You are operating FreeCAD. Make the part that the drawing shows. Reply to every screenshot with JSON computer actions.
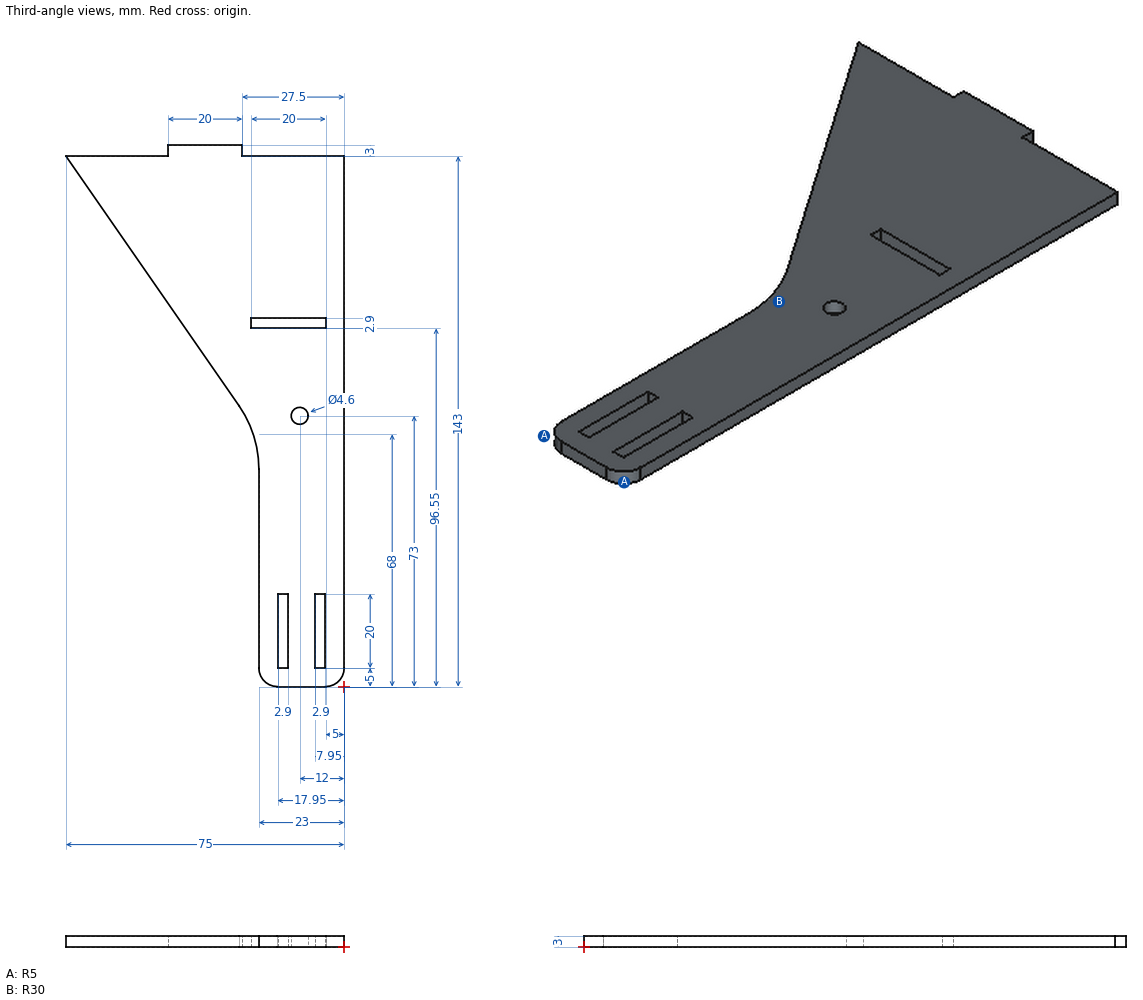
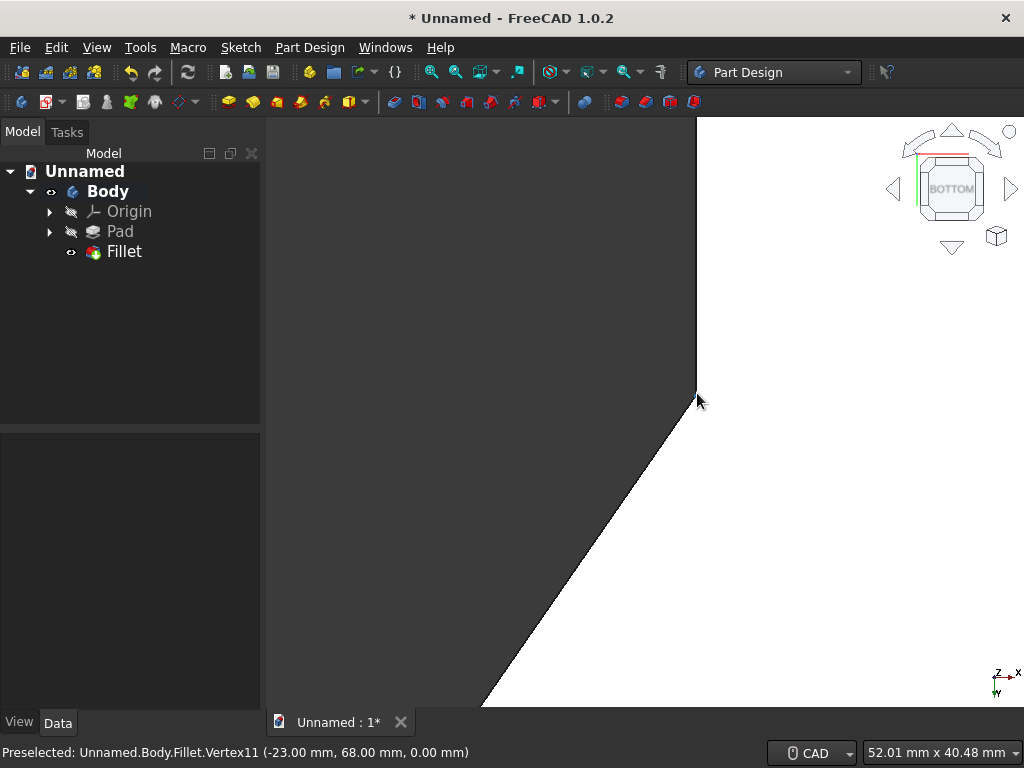
{"action": "key", "text": "v f"}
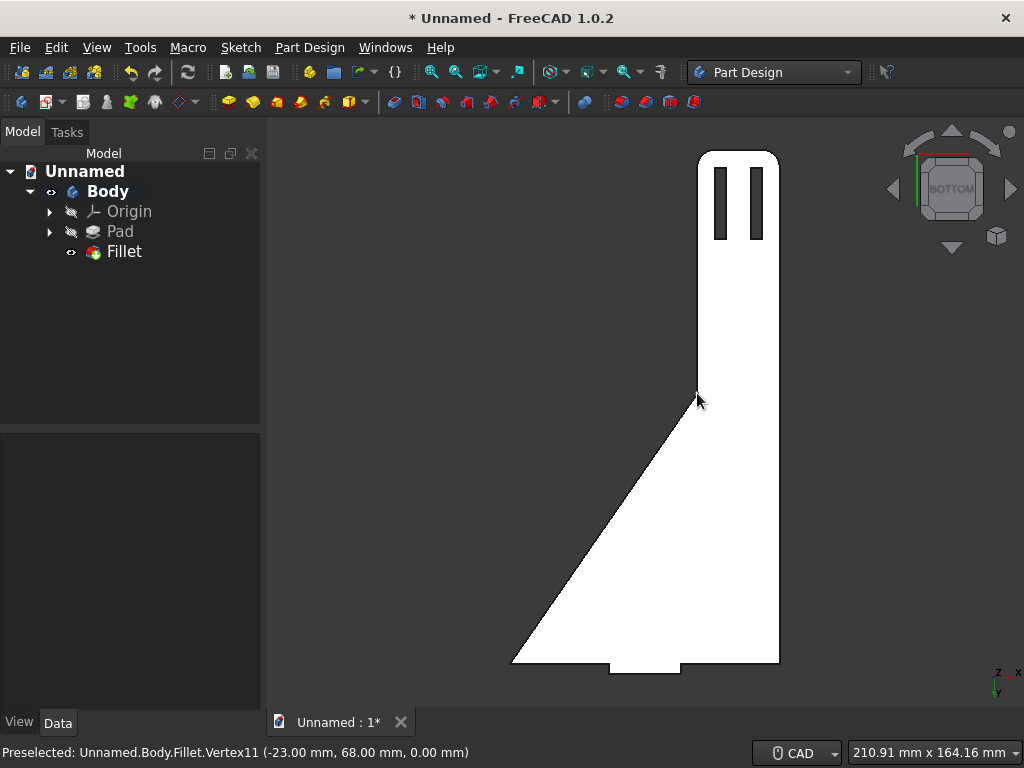
{"action": "key", "text": "4"}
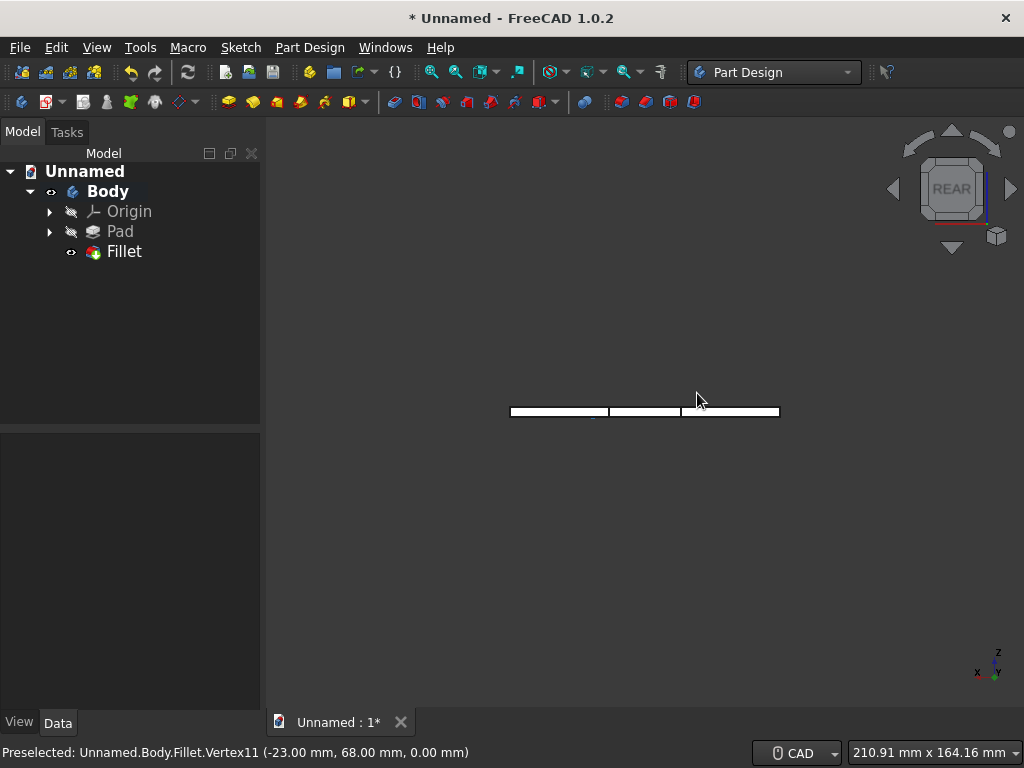
{"action": "left_click", "coordinate": [432, 72]}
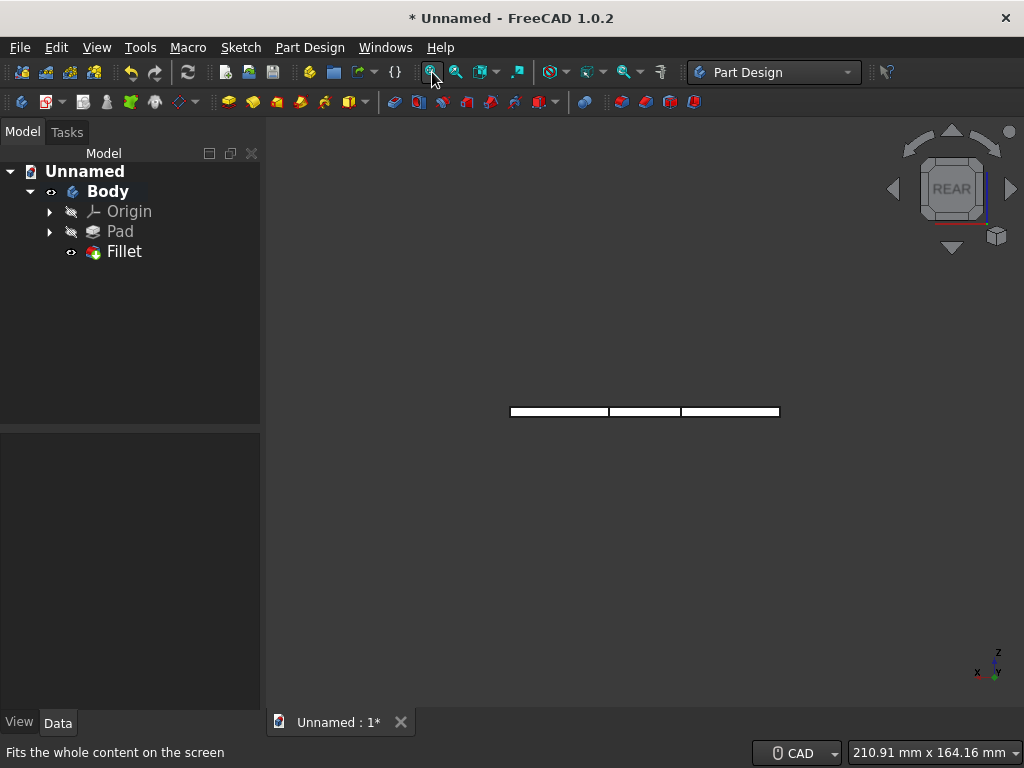
{"action": "scroll", "coordinate": [593, 411], "scroll_direction": "up", "scroll_amount": 7}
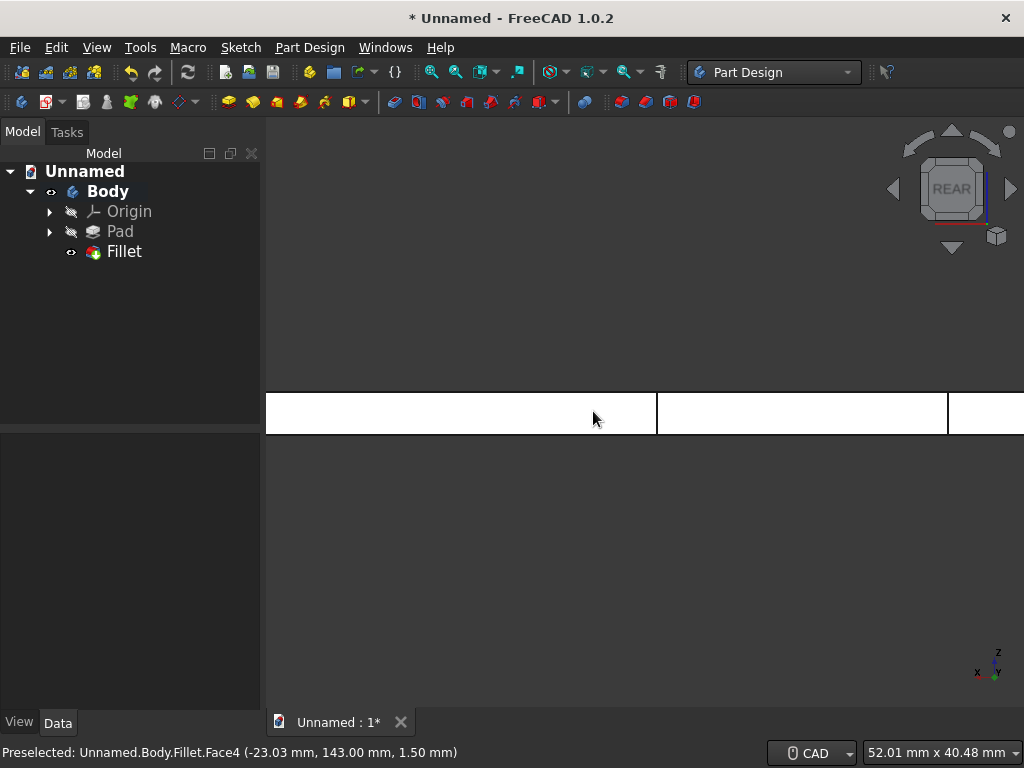
{"action": "left_click", "coordinate": [432, 72]}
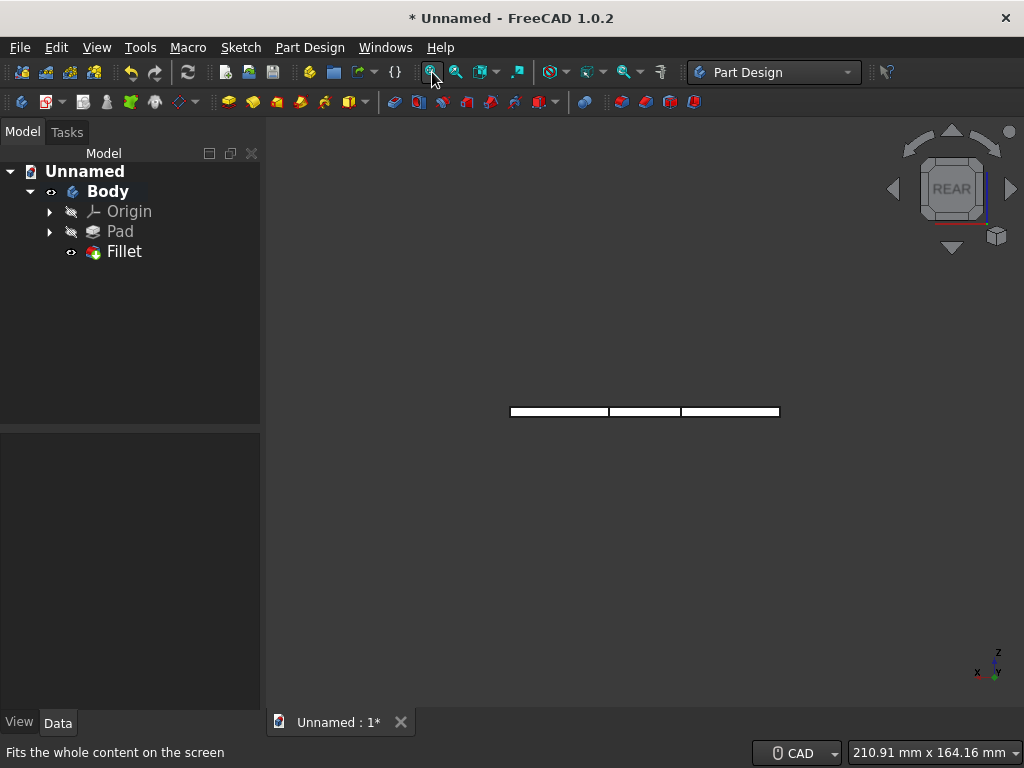
{"action": "key", "text": "6"}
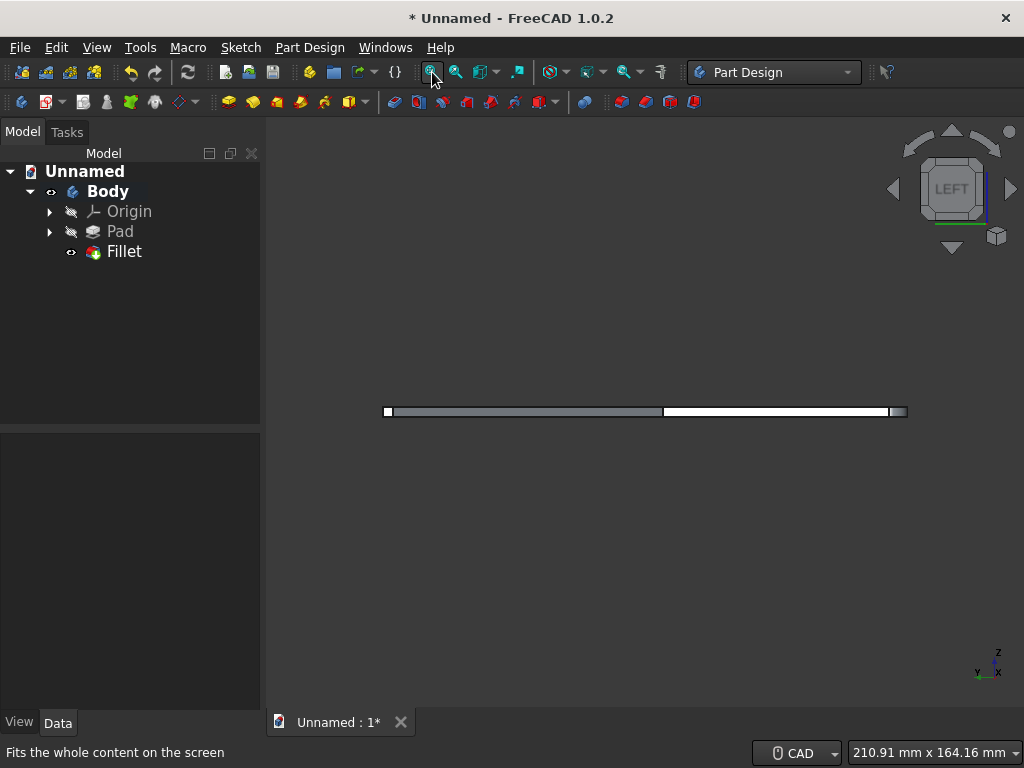
{"action": "scroll", "coordinate": [663, 411], "scroll_direction": "up", "scroll_amount": 7}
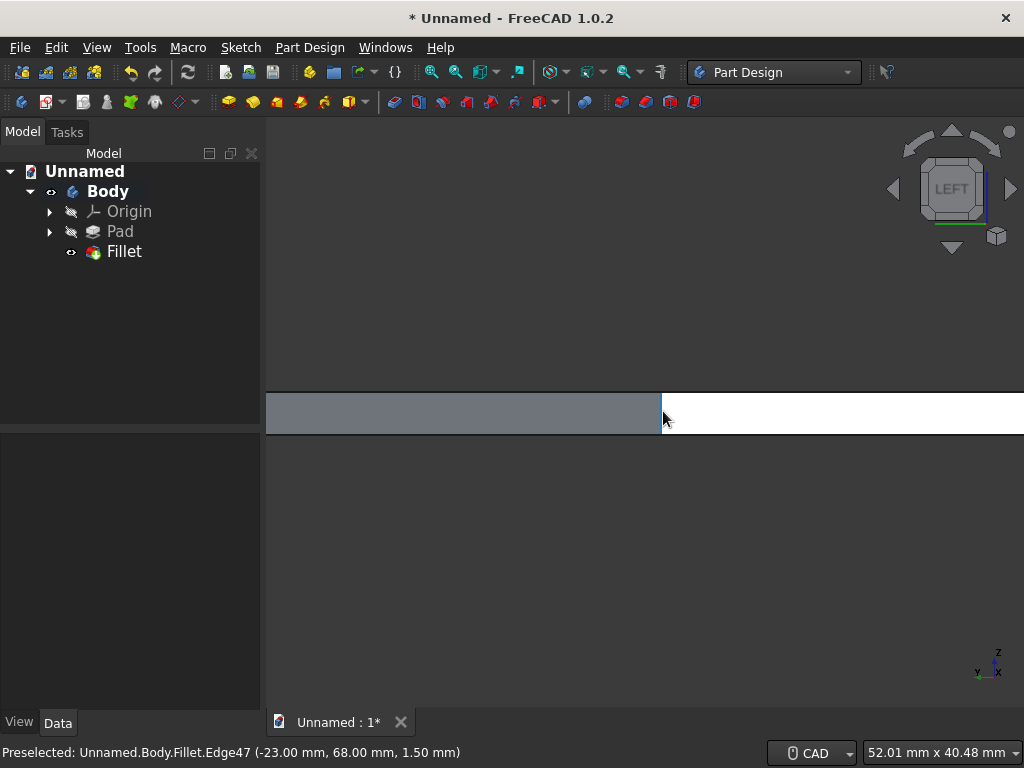
{"action": "key", "text": "v f"}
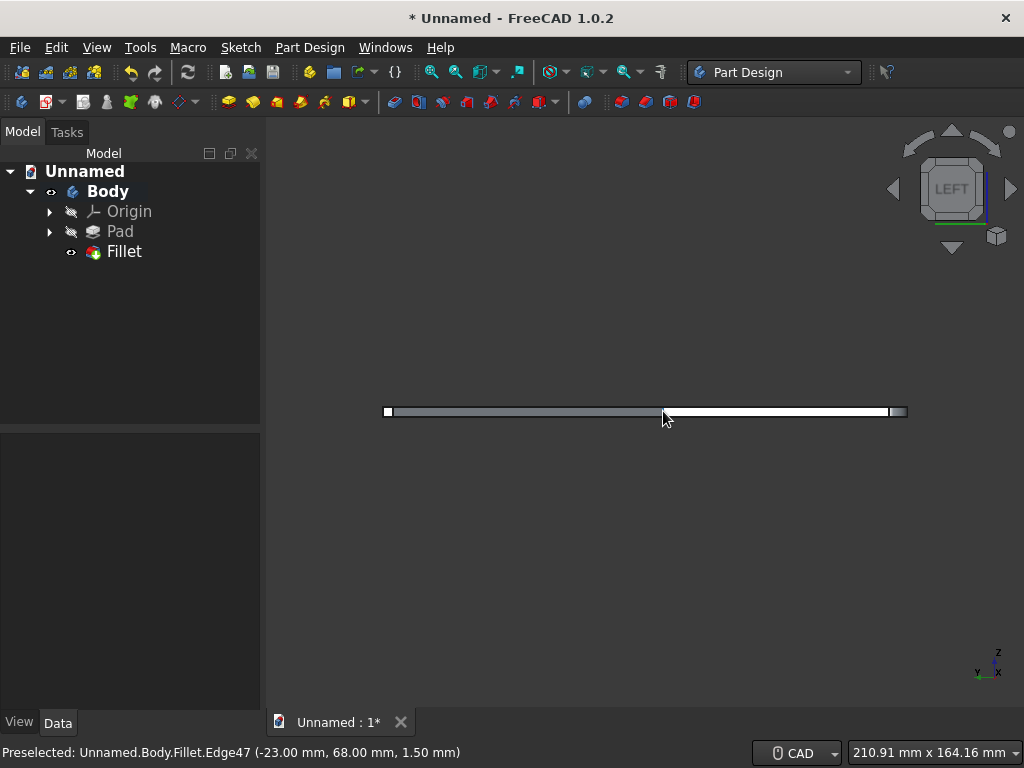
{"action": "key", "text": "v 3"}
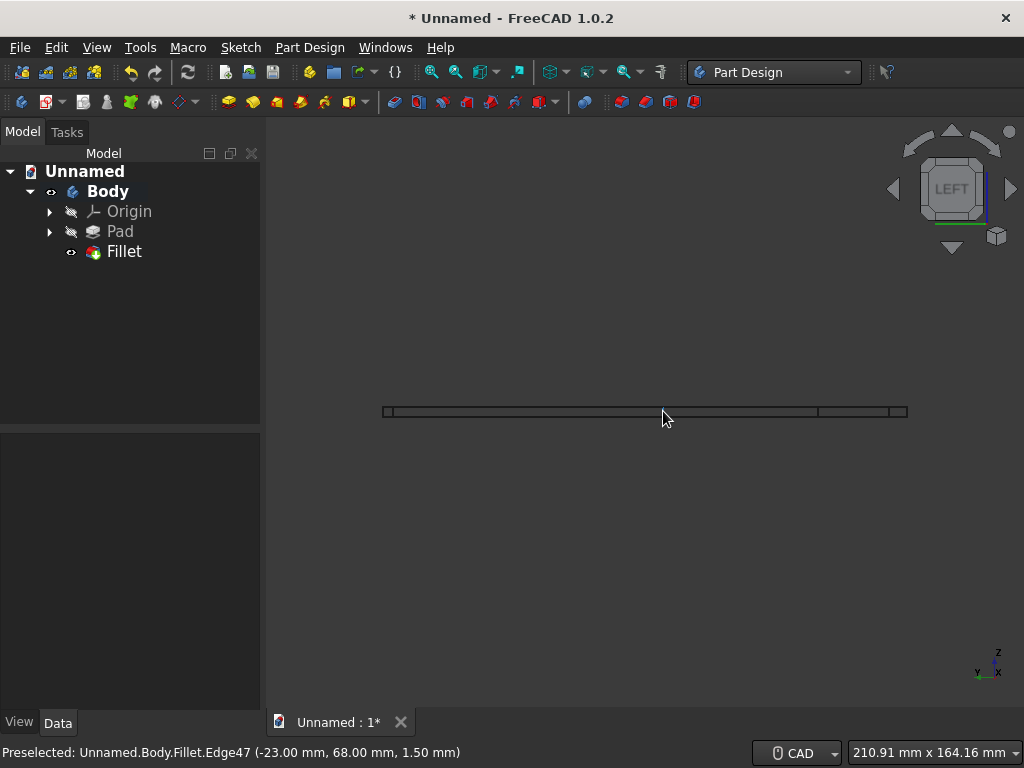
{"action": "key", "text": "0"}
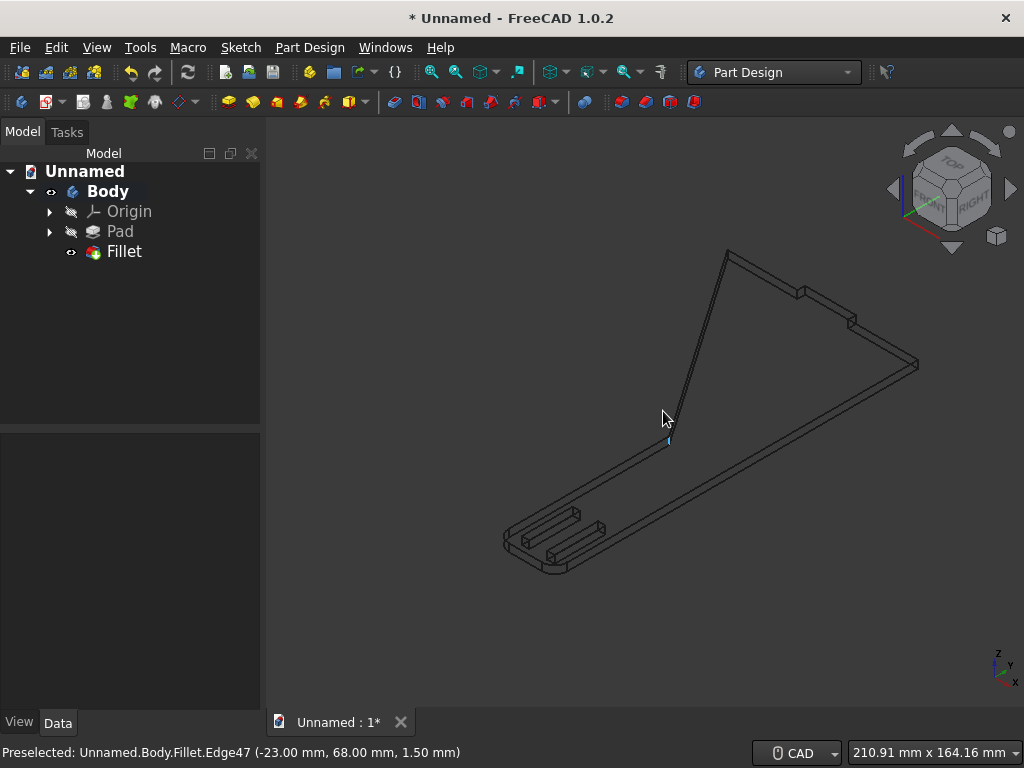
{"action": "scroll", "coordinate": [669, 440], "scroll_direction": "up", "scroll_amount": 7}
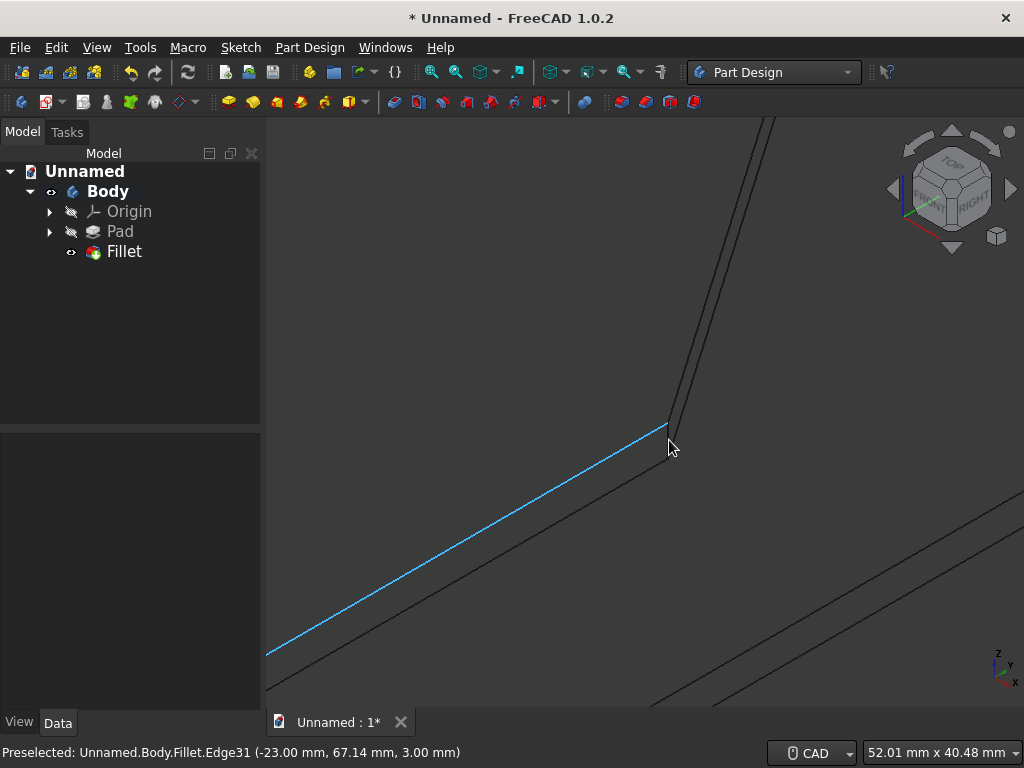
{"action": "left_click", "coordinate": [668, 440]}